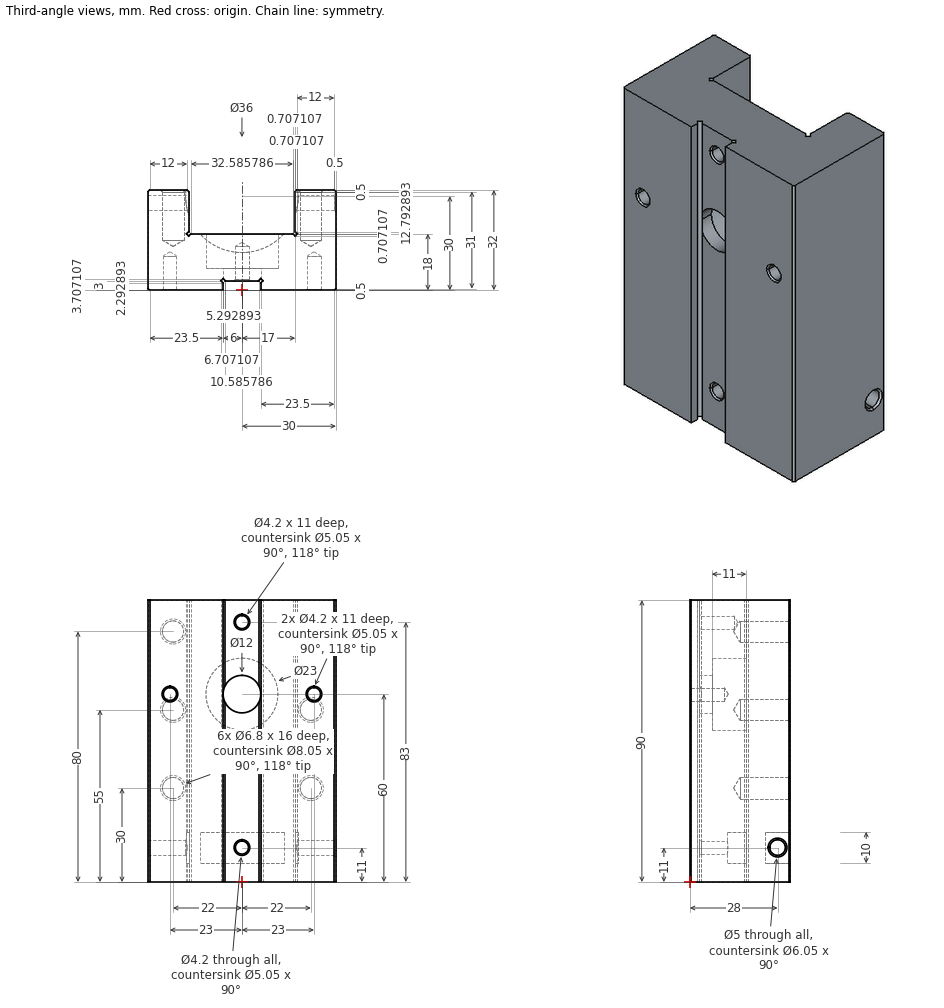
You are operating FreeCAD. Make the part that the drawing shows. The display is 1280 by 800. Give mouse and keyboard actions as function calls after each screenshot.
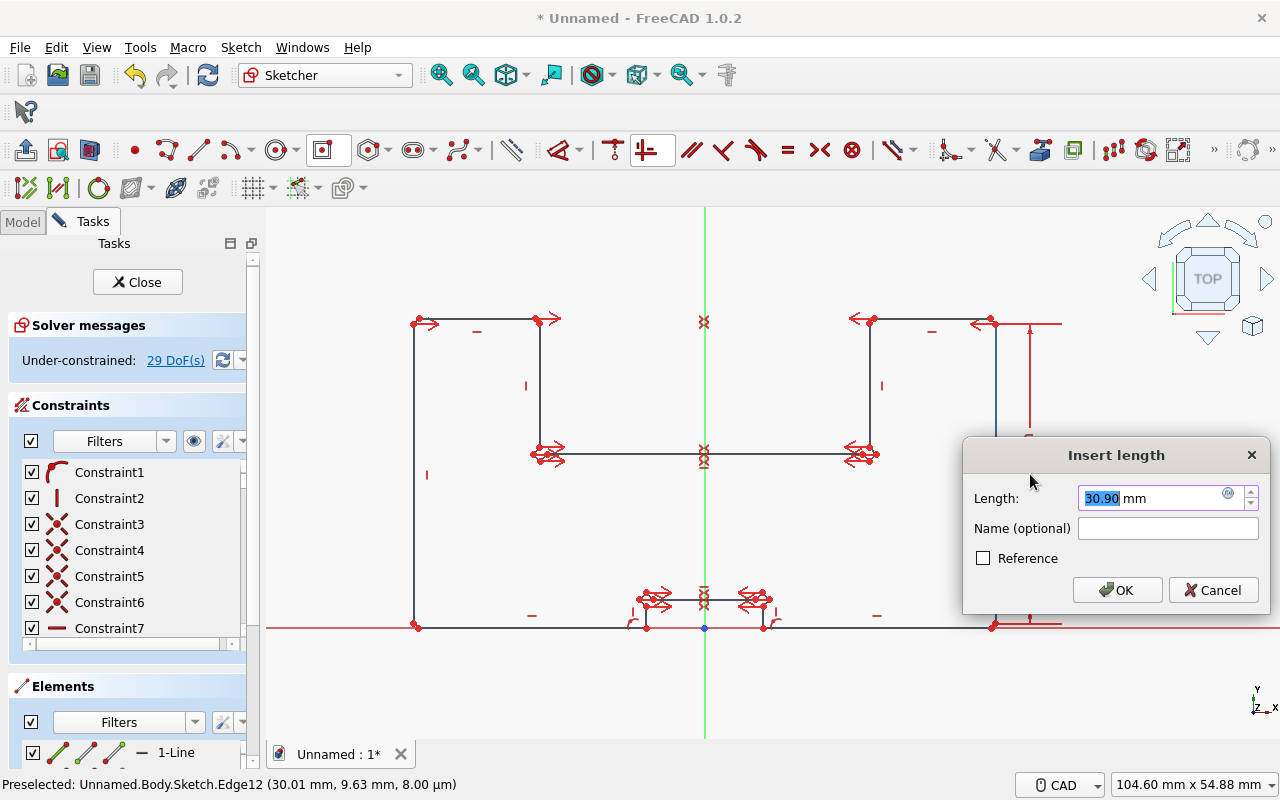
text(31)
key(Return)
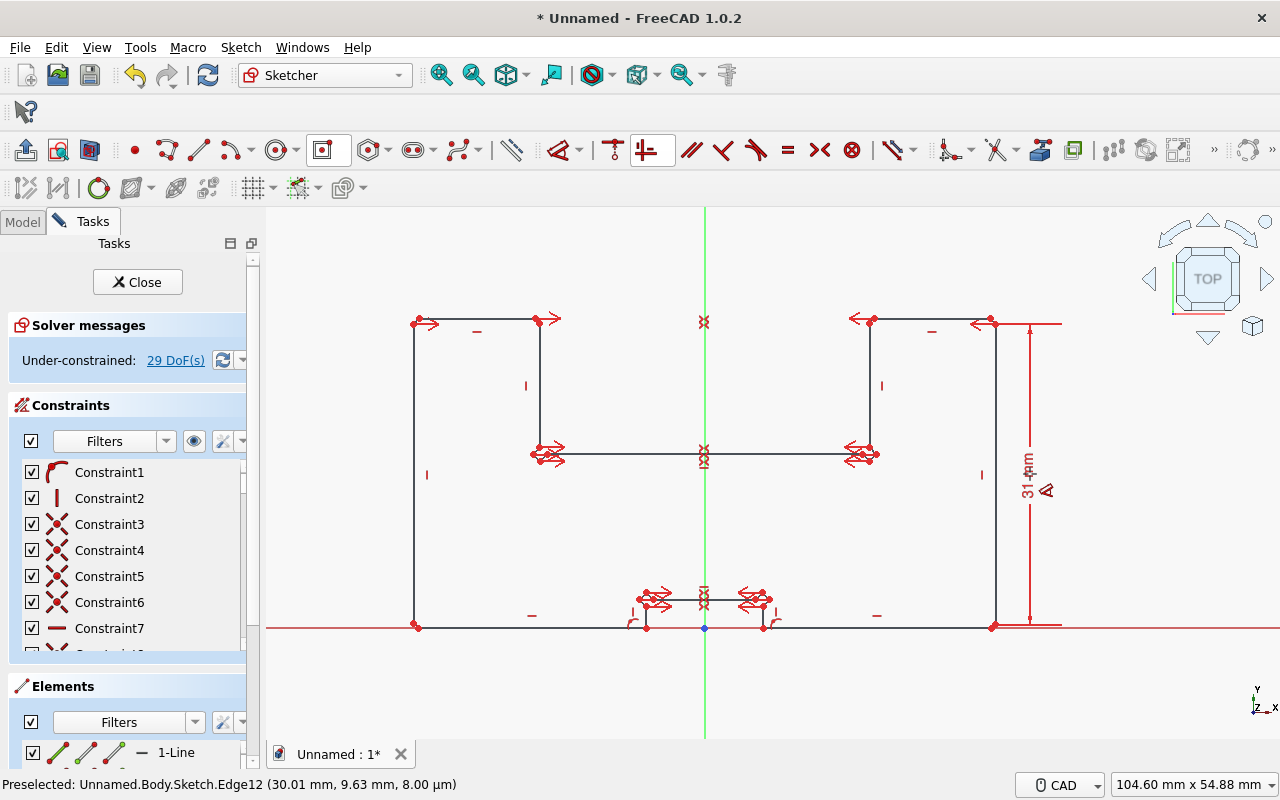
click(956, 318)
click(933, 284)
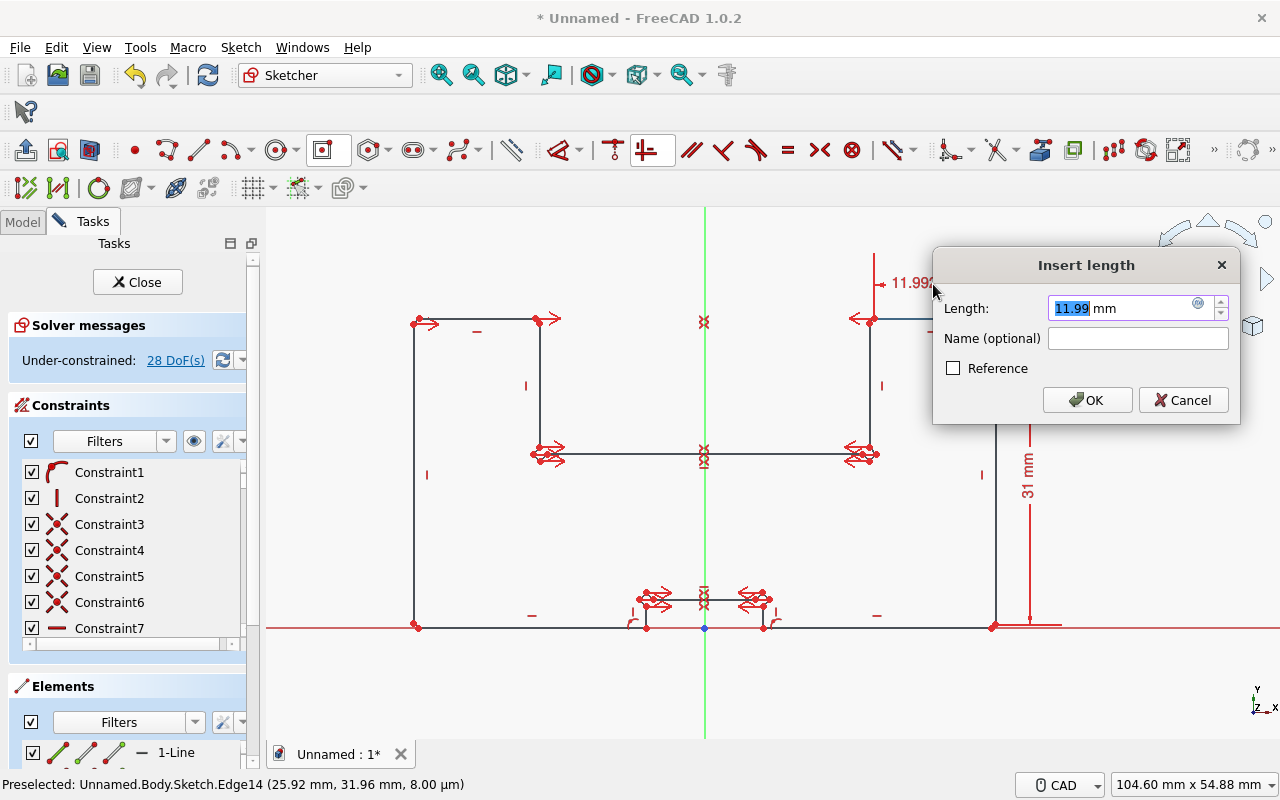
text(12)
key(Return)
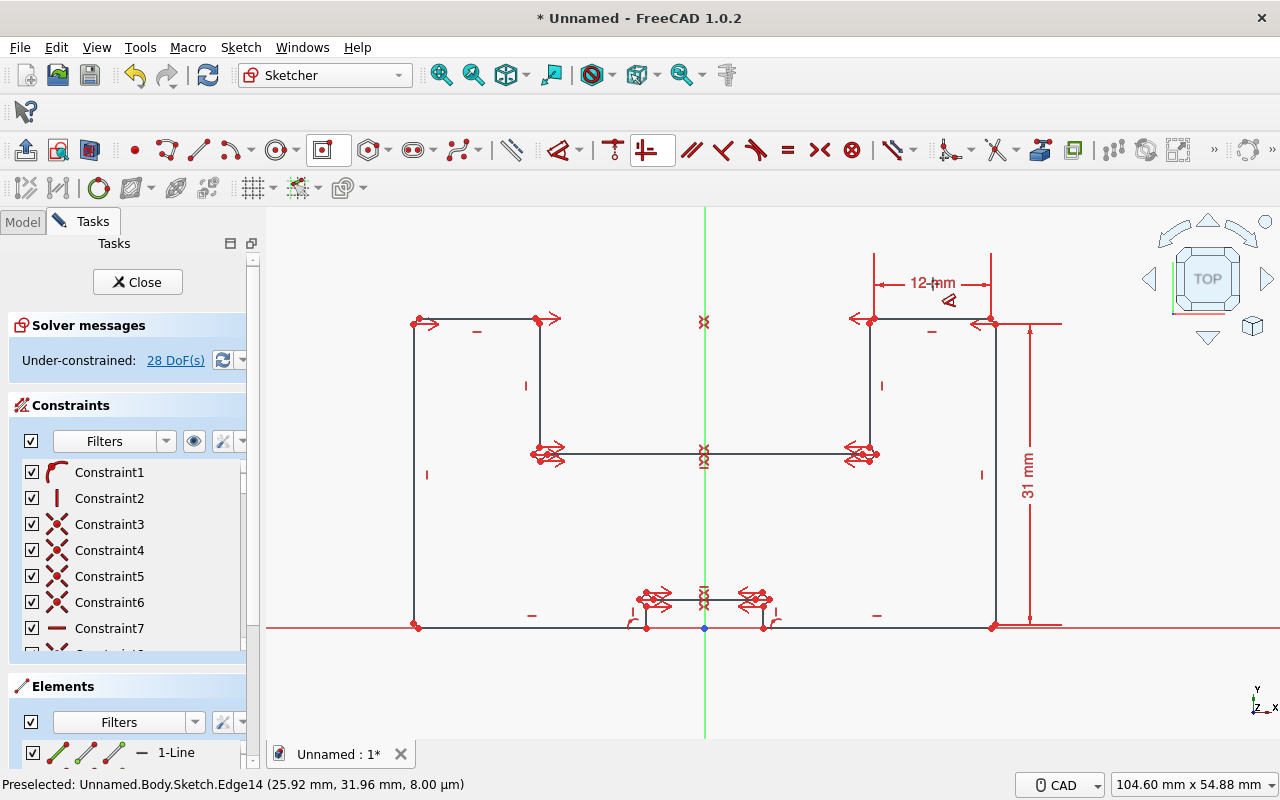
click(500, 318)
click(477, 284)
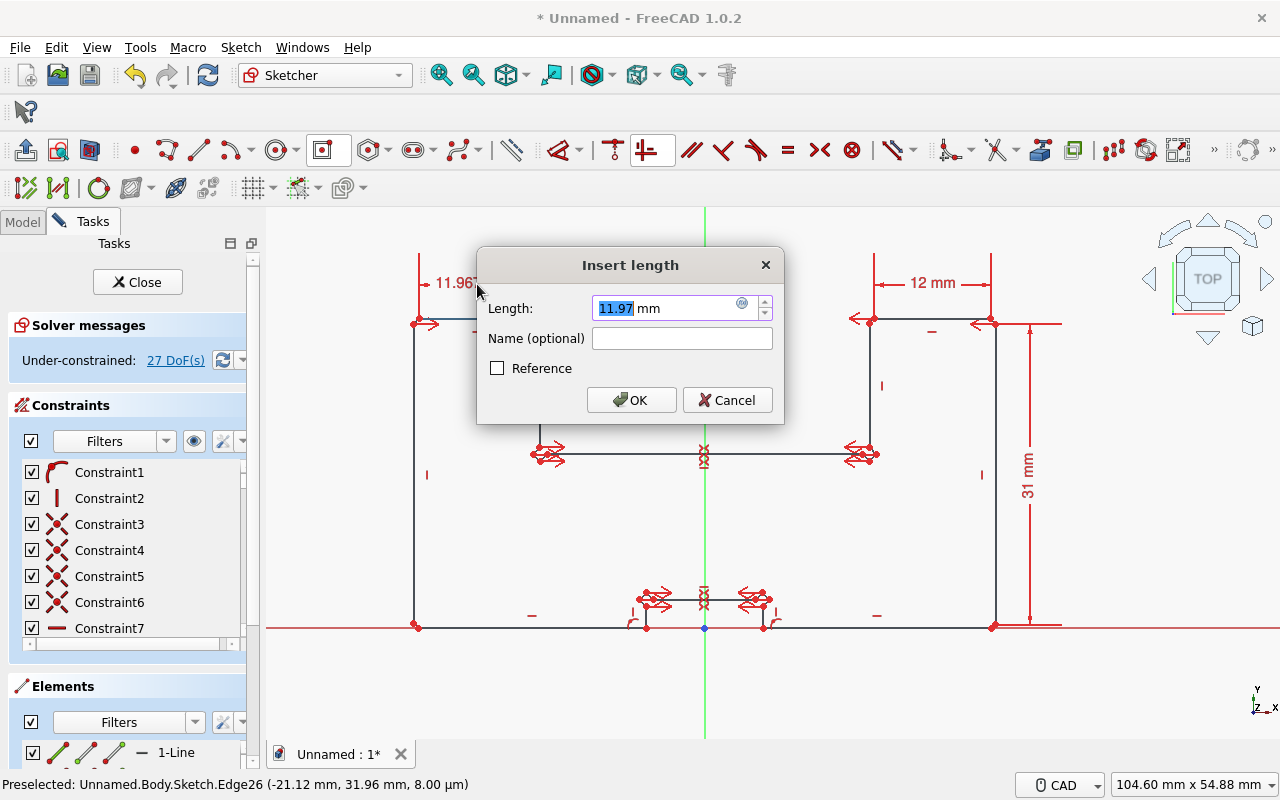
text(12)
key(Return)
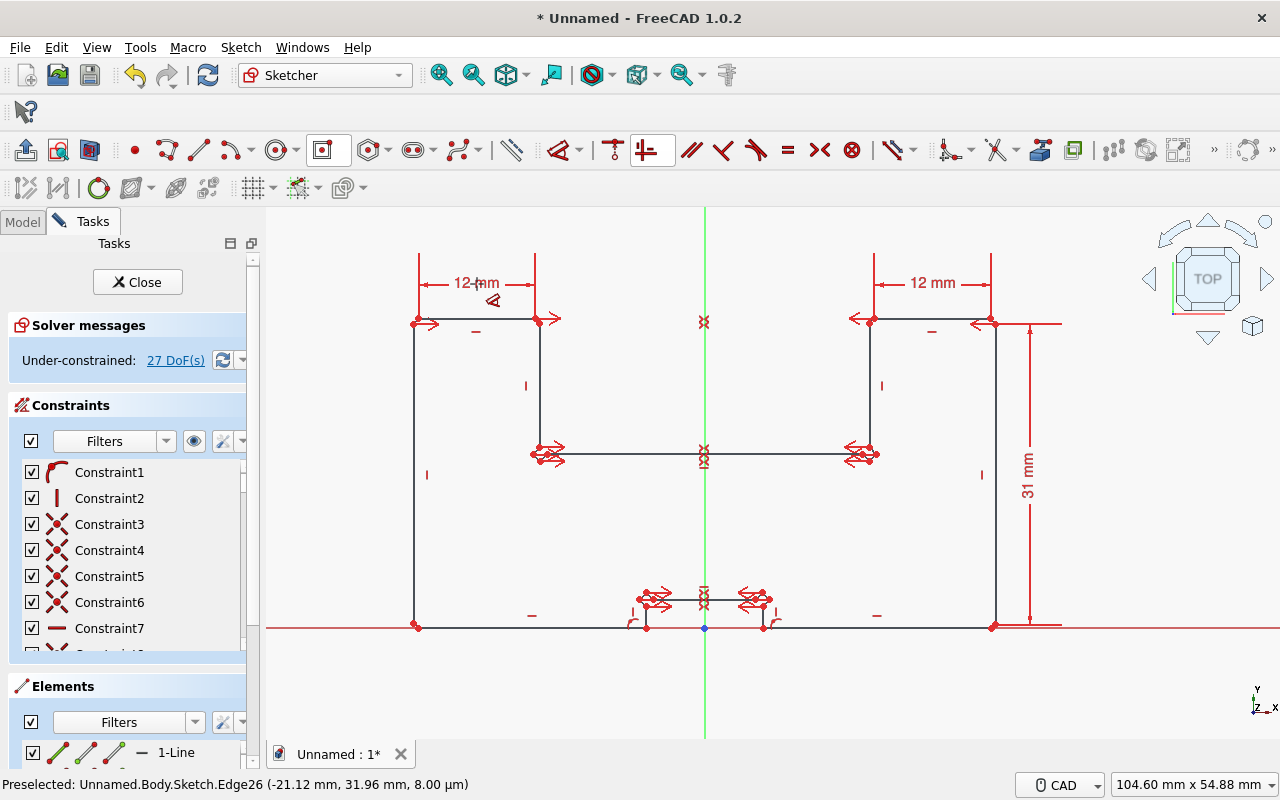
click(414, 414)
click(380, 474)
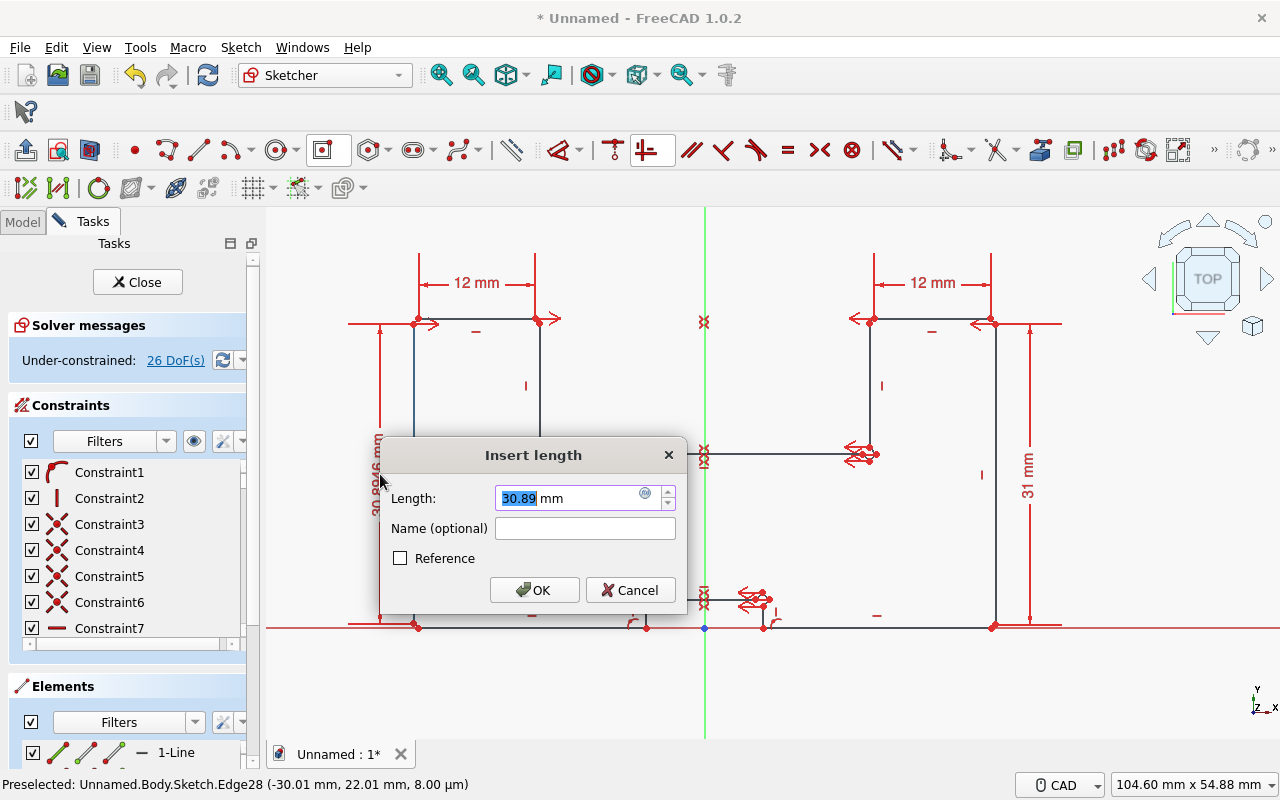
text(31)
key(Return)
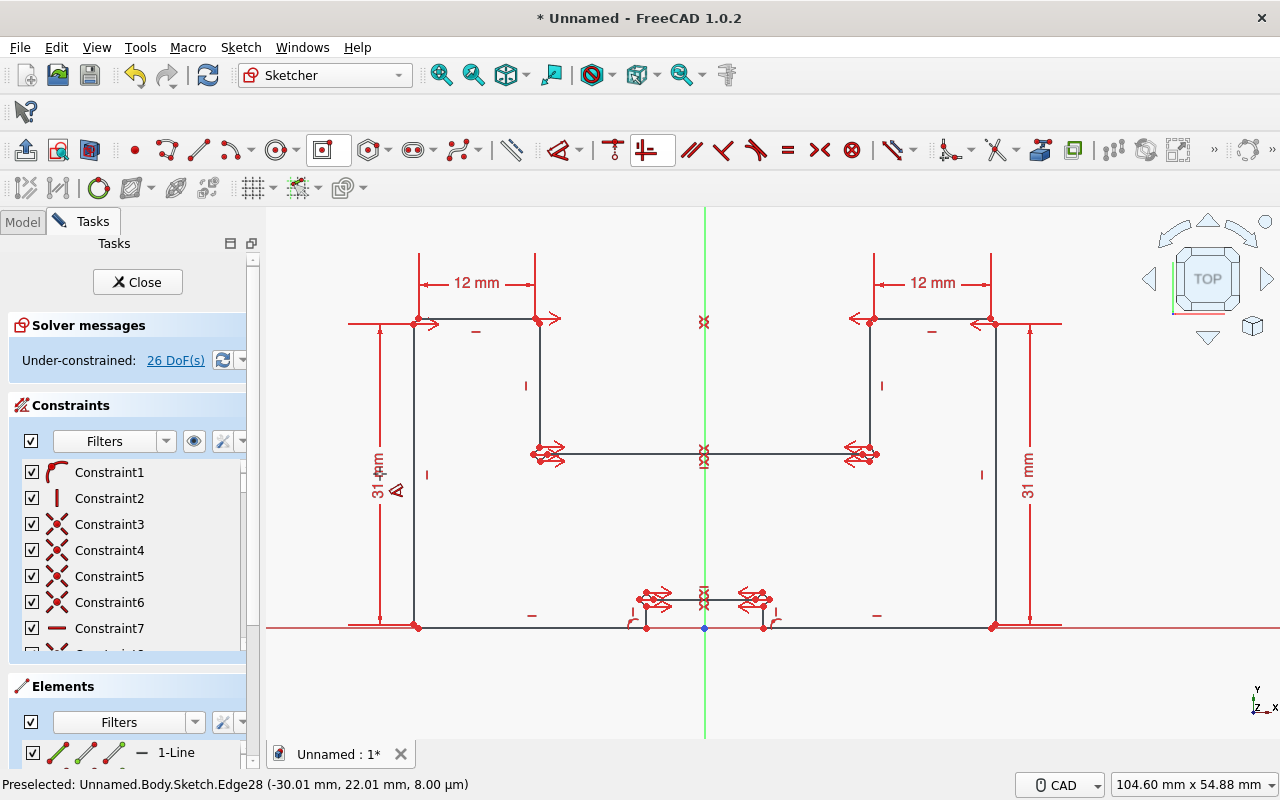
click(646, 628)
click(676, 662)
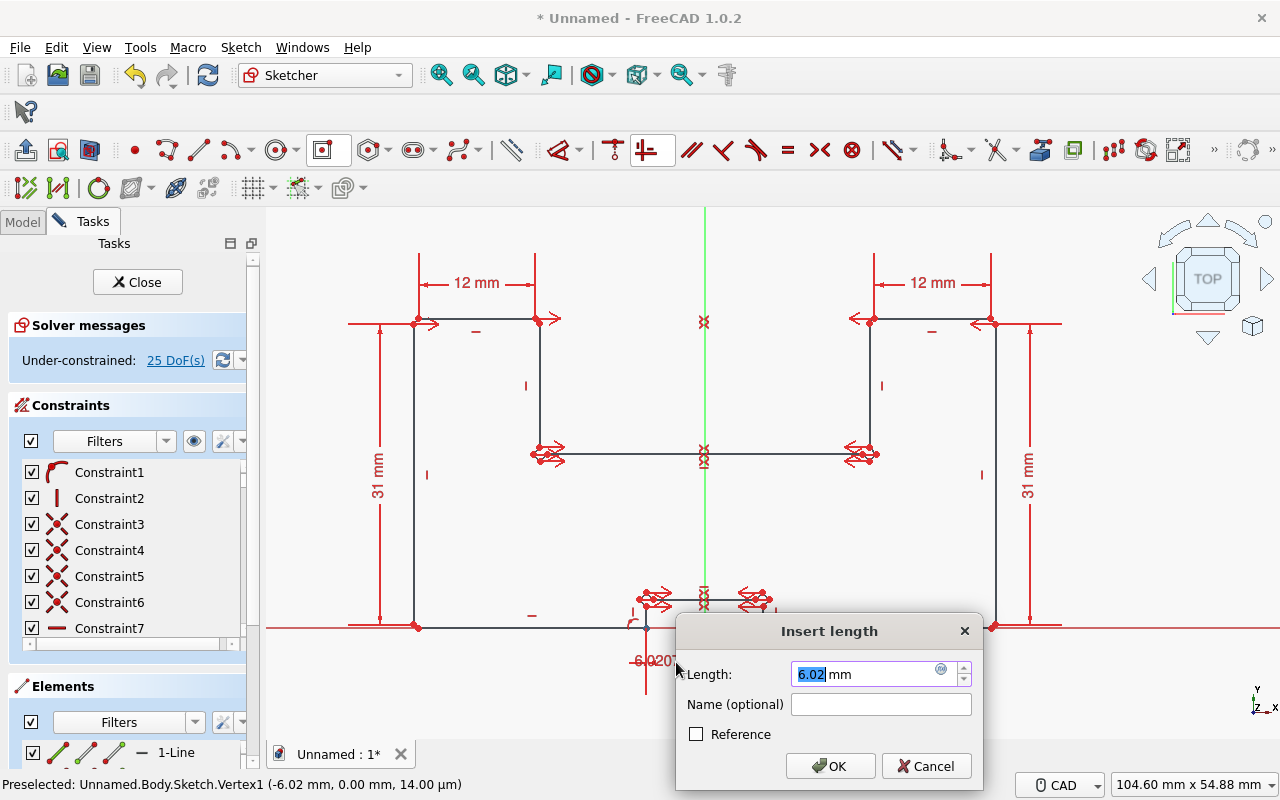
text(6)
key(Return)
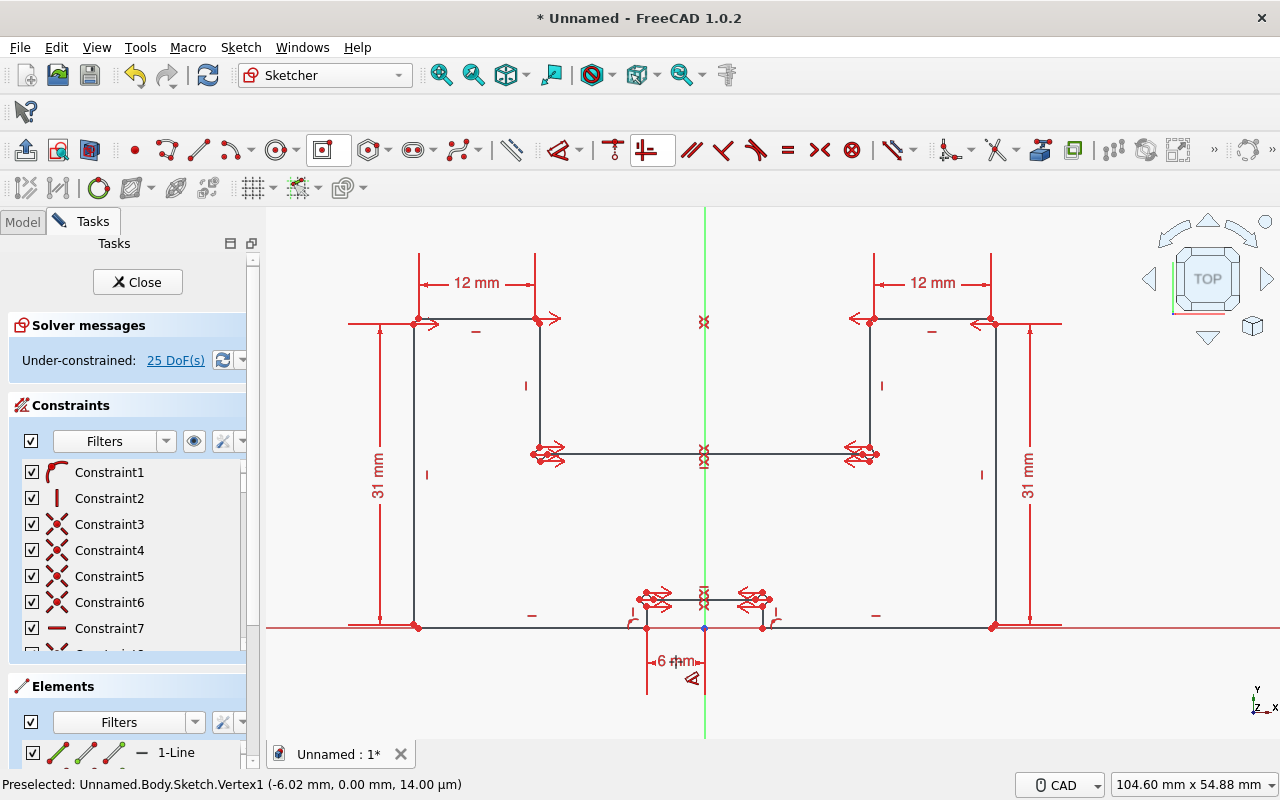
scroll(640, 600, up, 2)